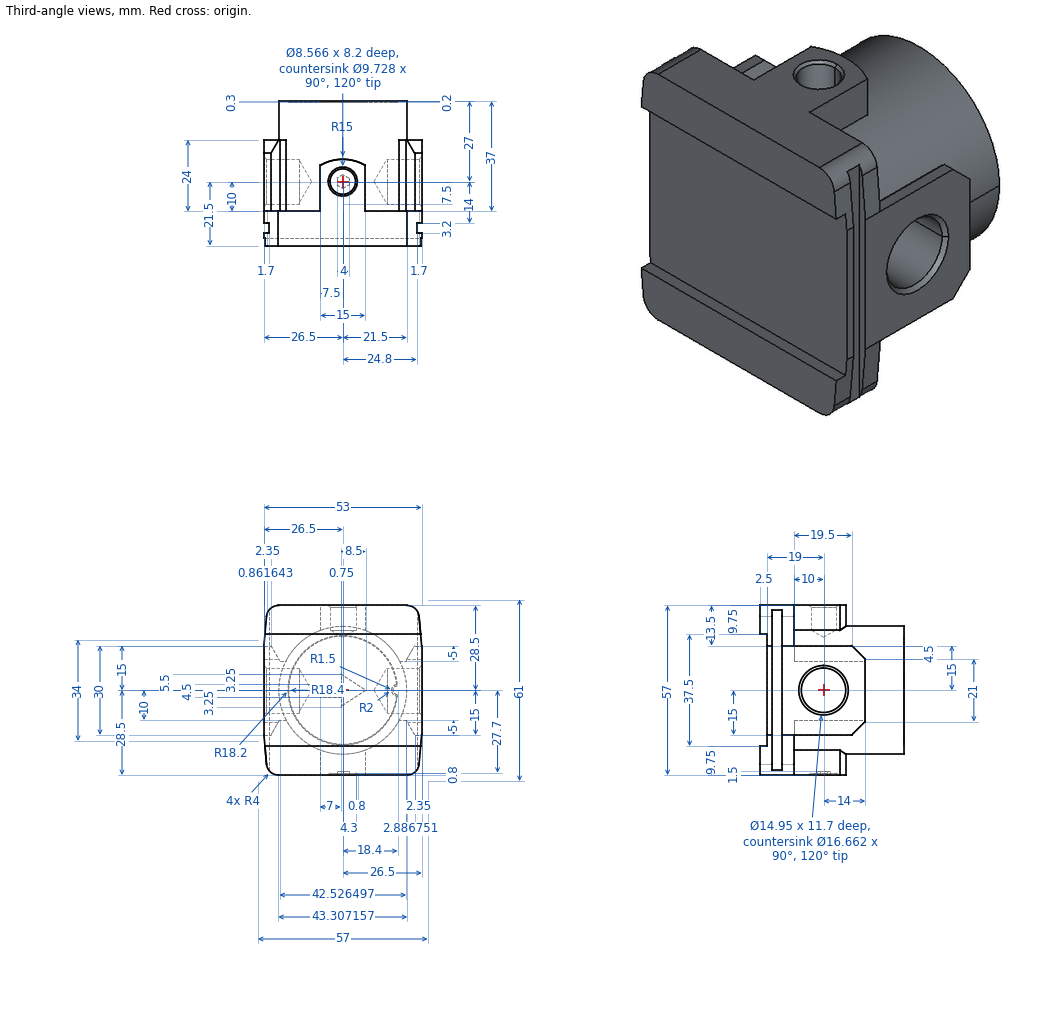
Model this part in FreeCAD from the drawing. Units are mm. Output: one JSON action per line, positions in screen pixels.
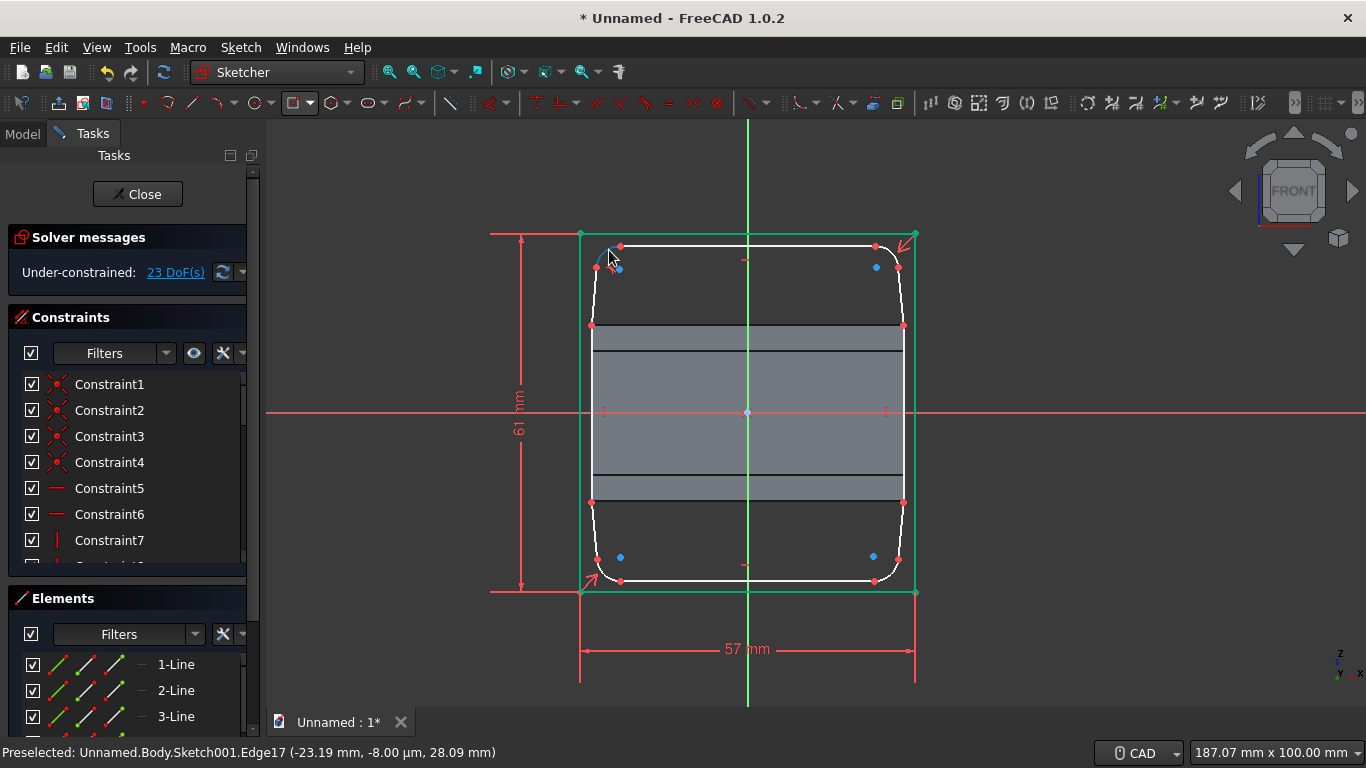
{"action": "left_click", "coordinate": [593, 519]}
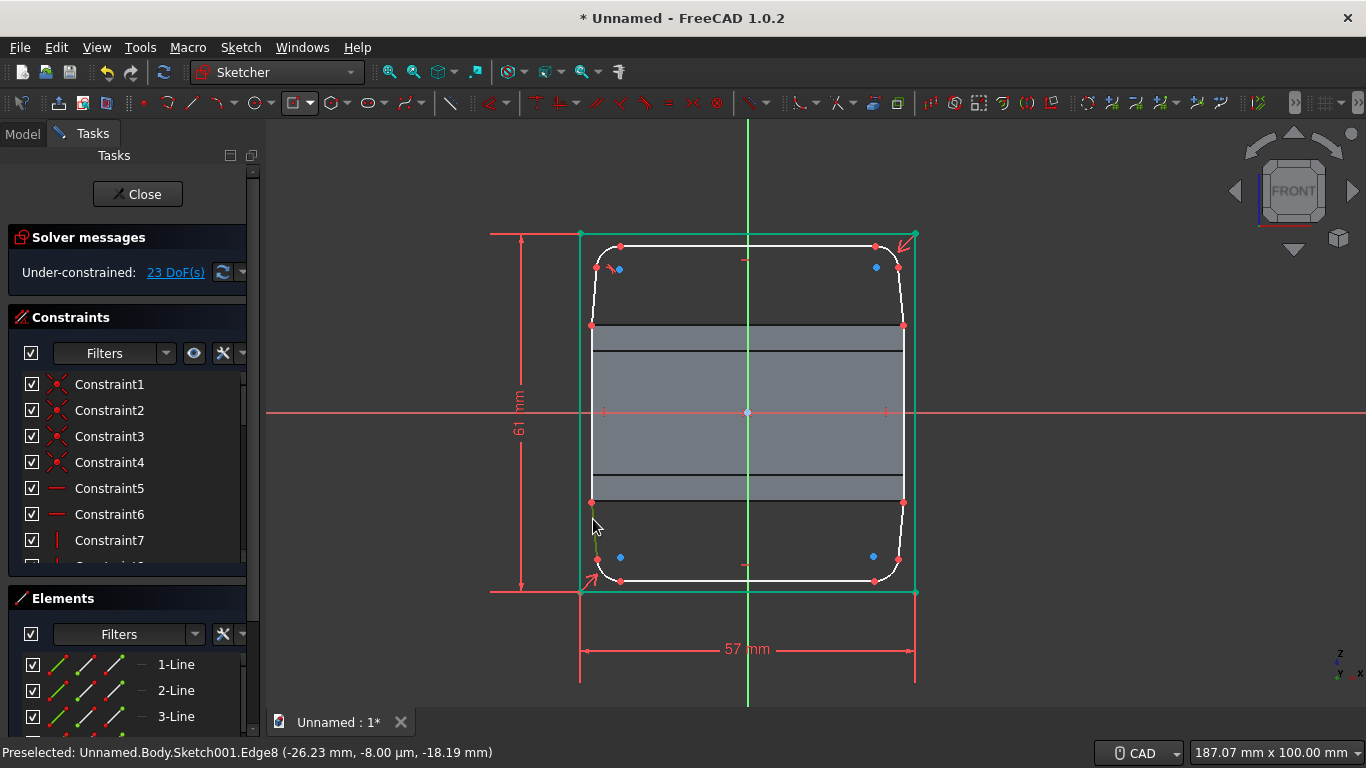
{"action": "scroll", "coordinate": [600, 570], "scroll_direction": "up", "scroll_amount": 2}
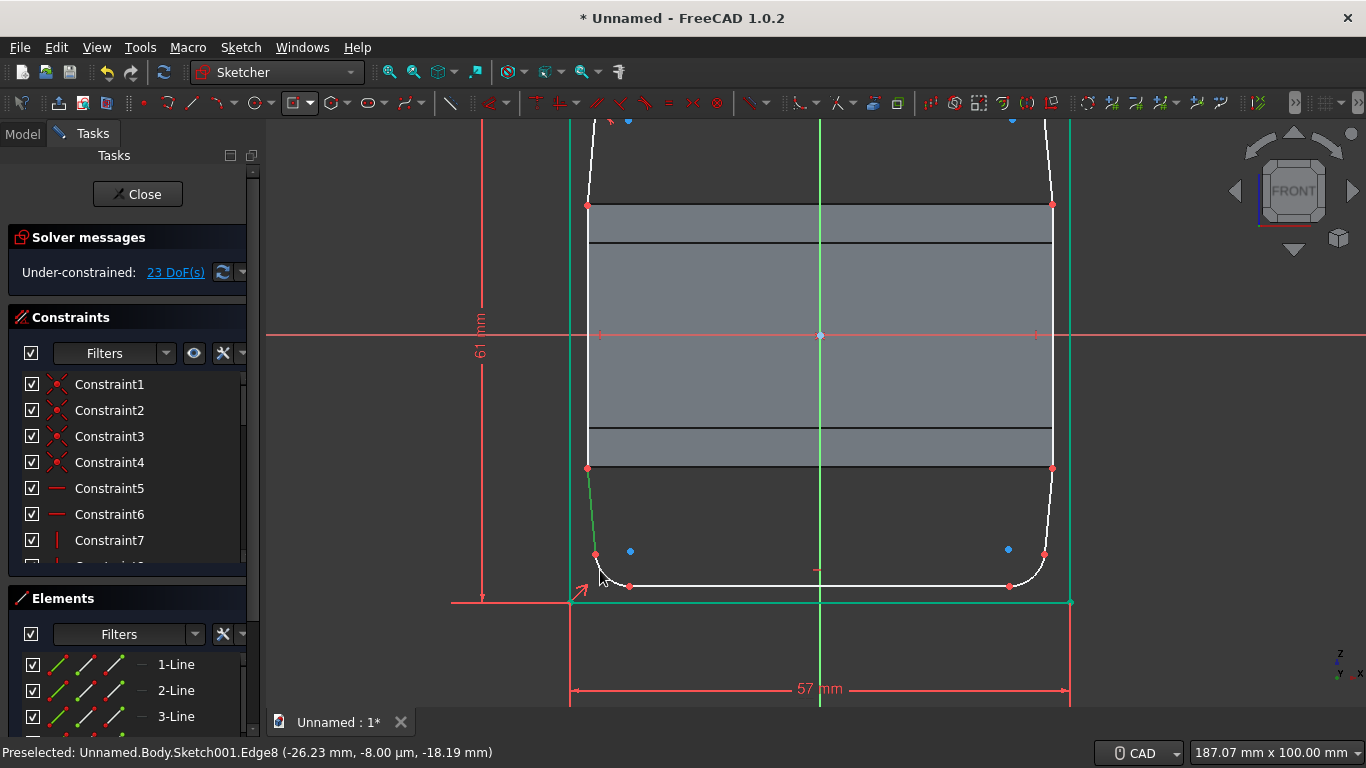
{"action": "left_click", "coordinate": [600, 569]}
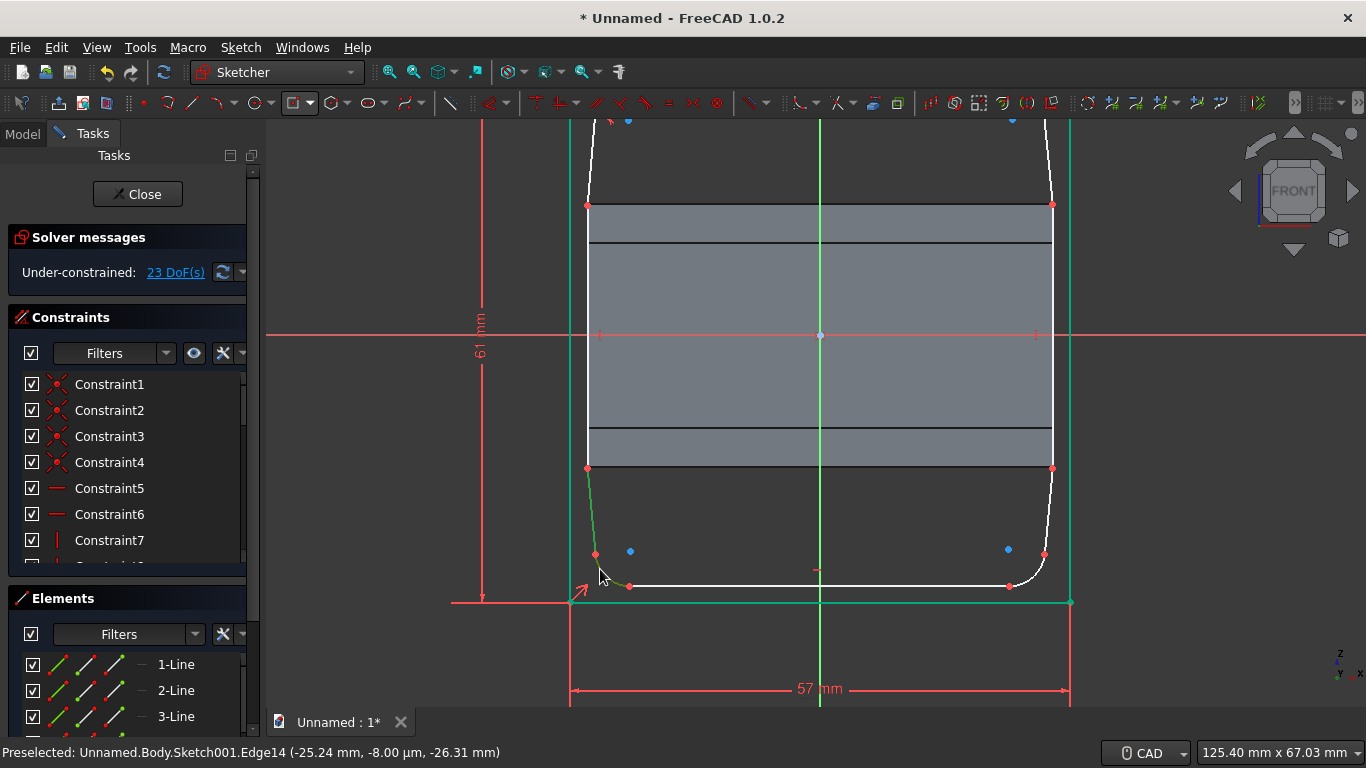
{"action": "left_click", "coordinate": [646, 104]}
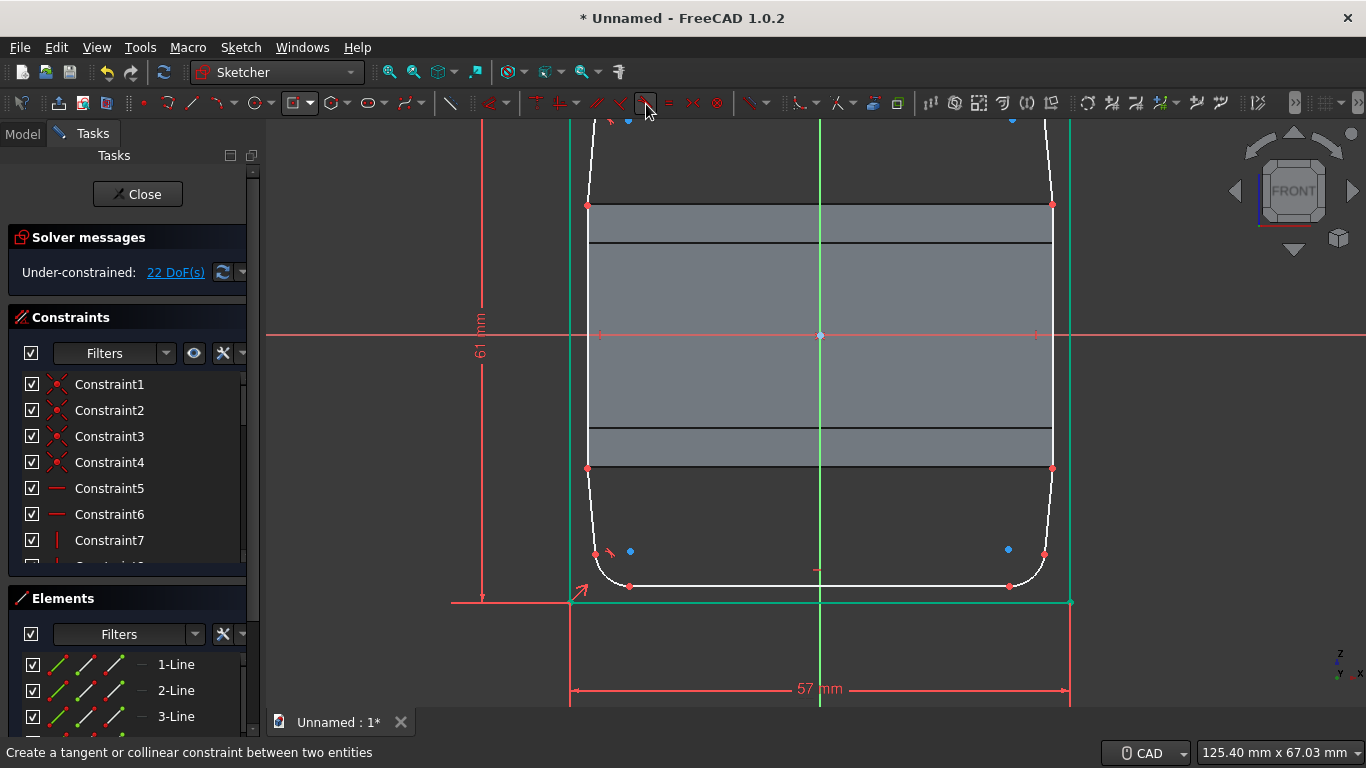
{"action": "left_click", "coordinate": [744, 586]}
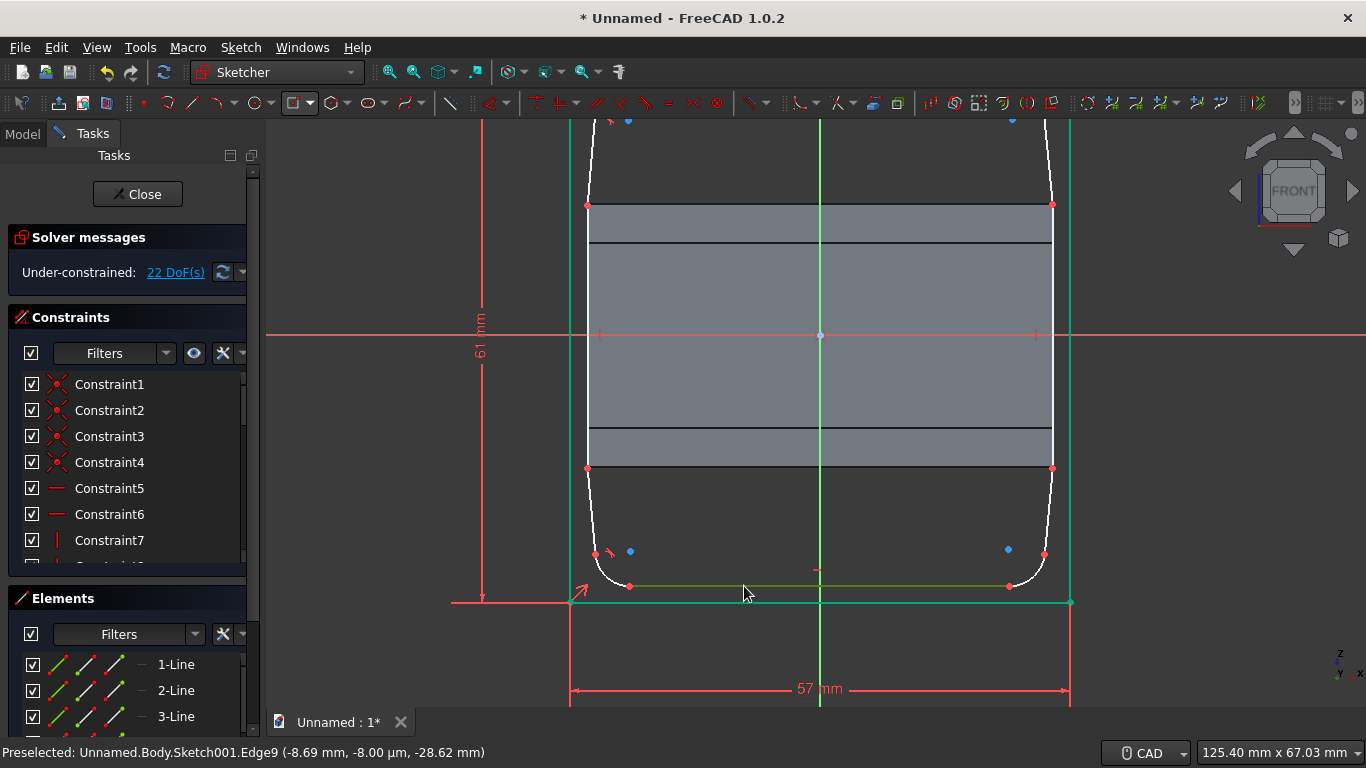
{"action": "left_click", "coordinate": [600, 569]}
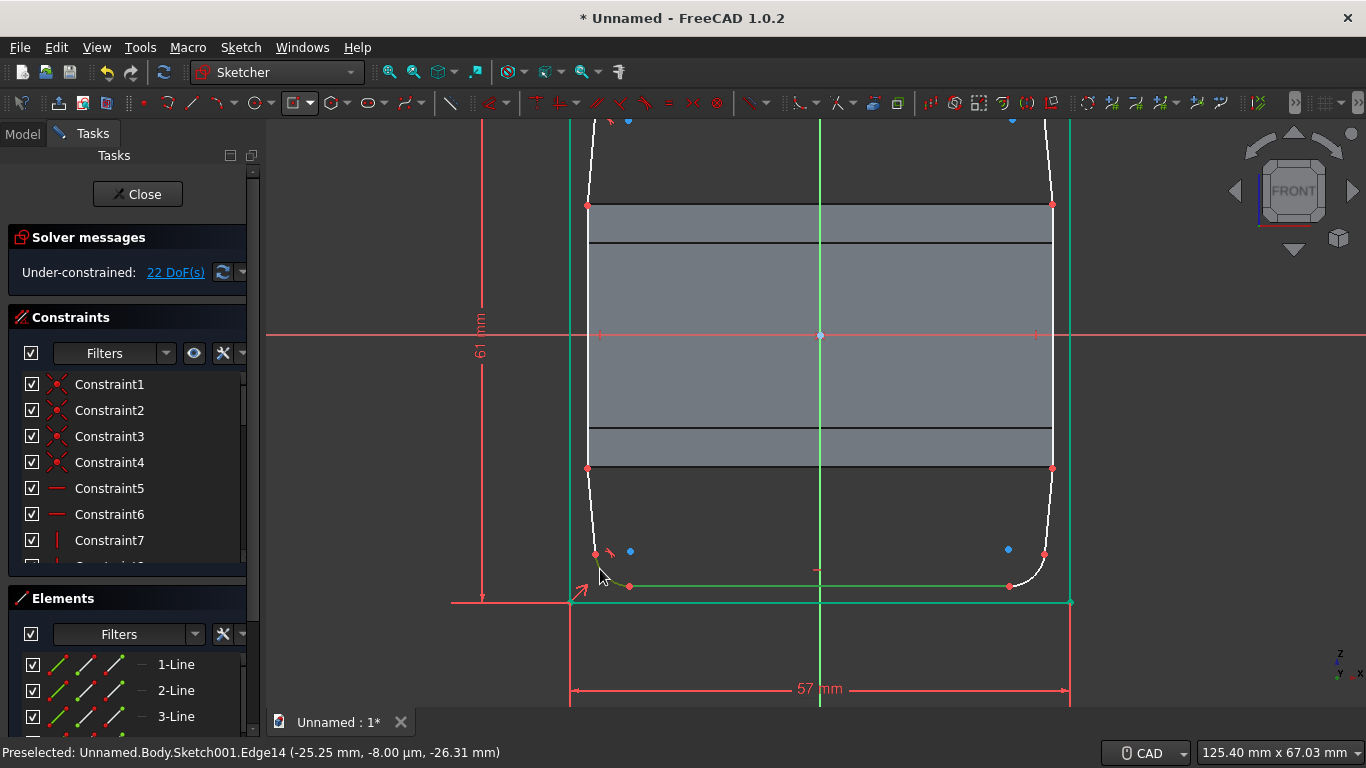
{"action": "key", "text": "t"}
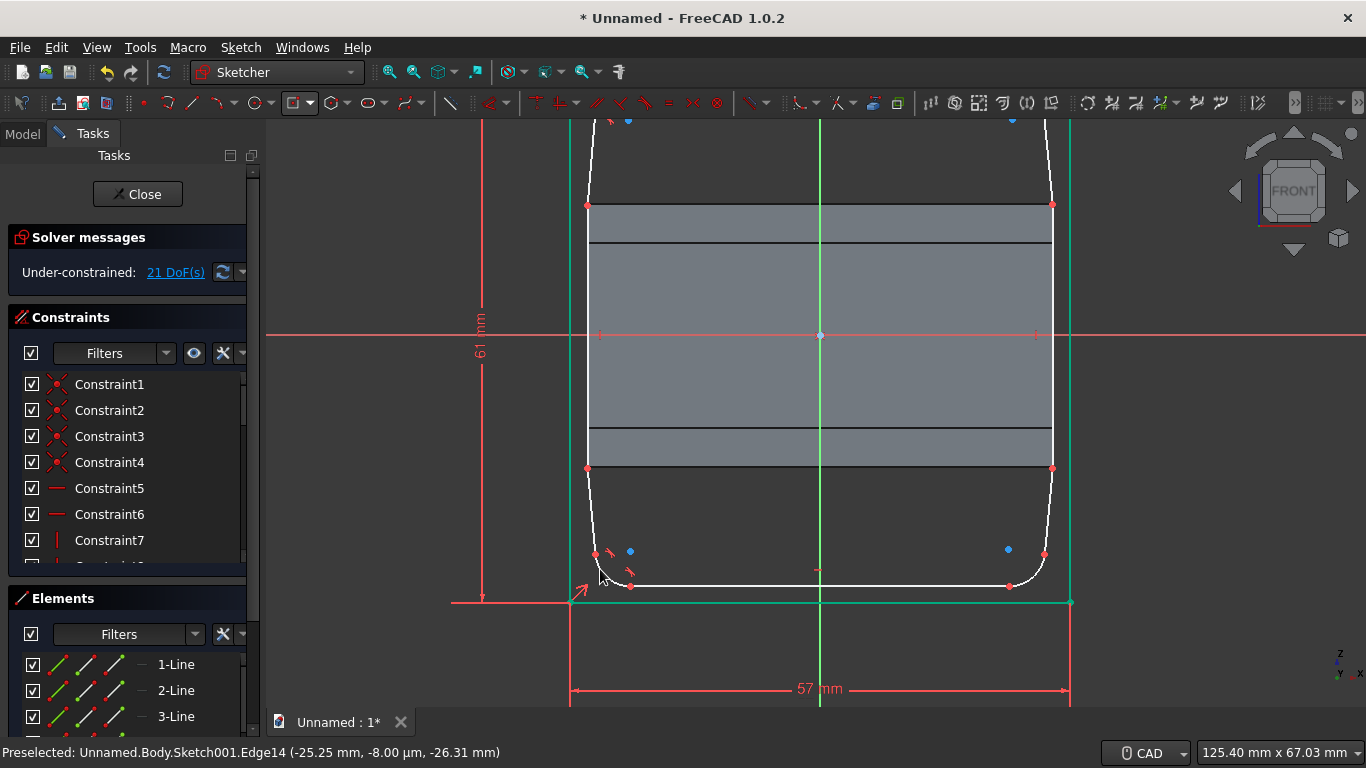
{"action": "left_click", "coordinate": [744, 586]}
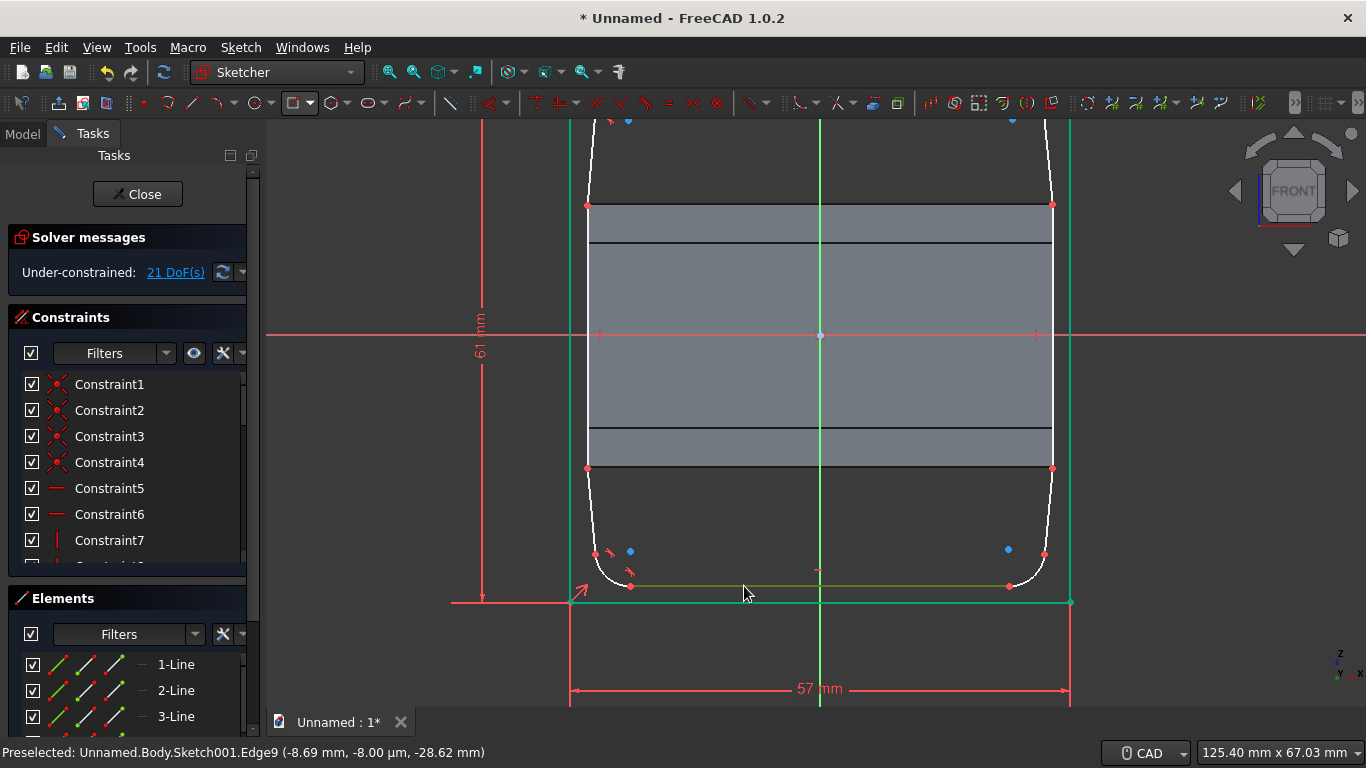
{"action": "left_click", "coordinate": [1025, 583]}